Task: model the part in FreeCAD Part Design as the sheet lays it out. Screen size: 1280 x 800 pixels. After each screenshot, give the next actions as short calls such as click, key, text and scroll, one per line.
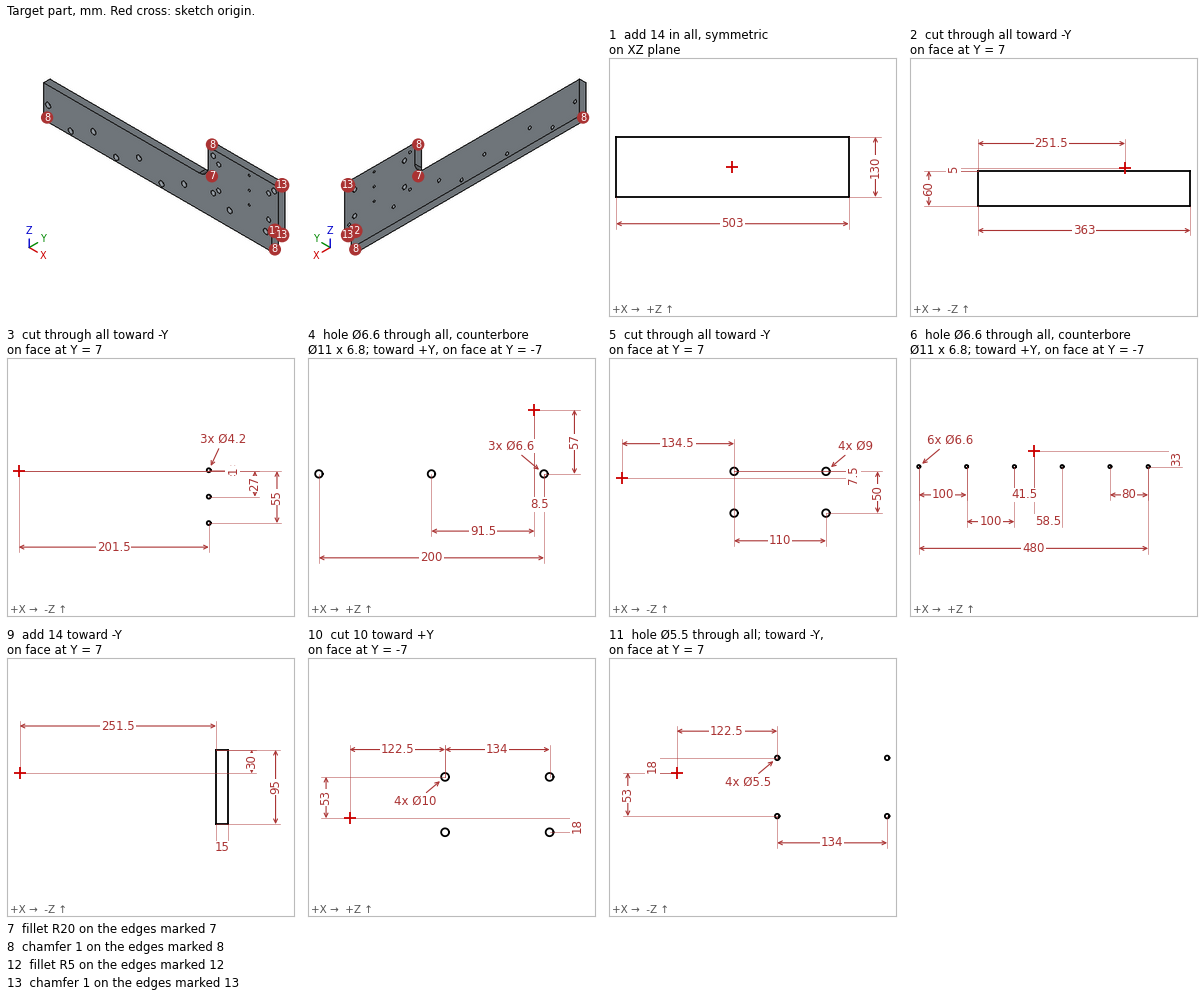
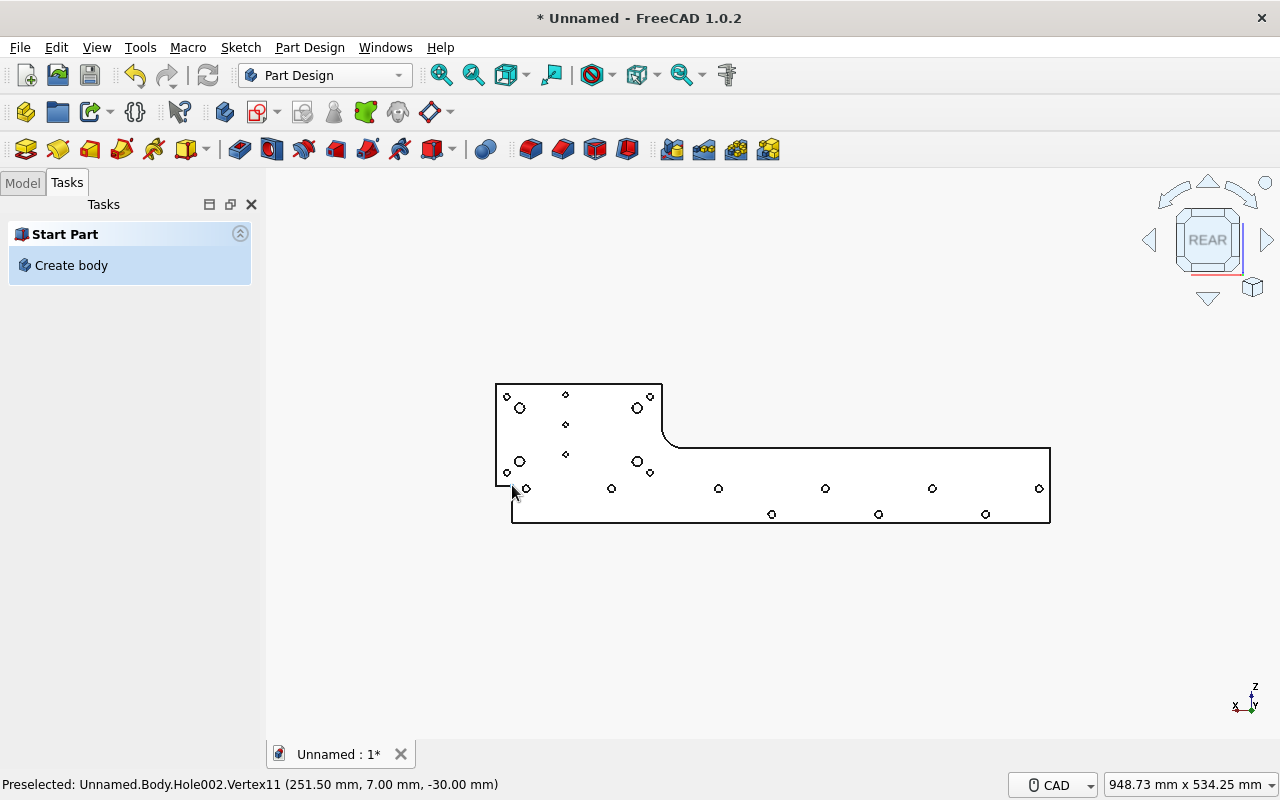
key(6)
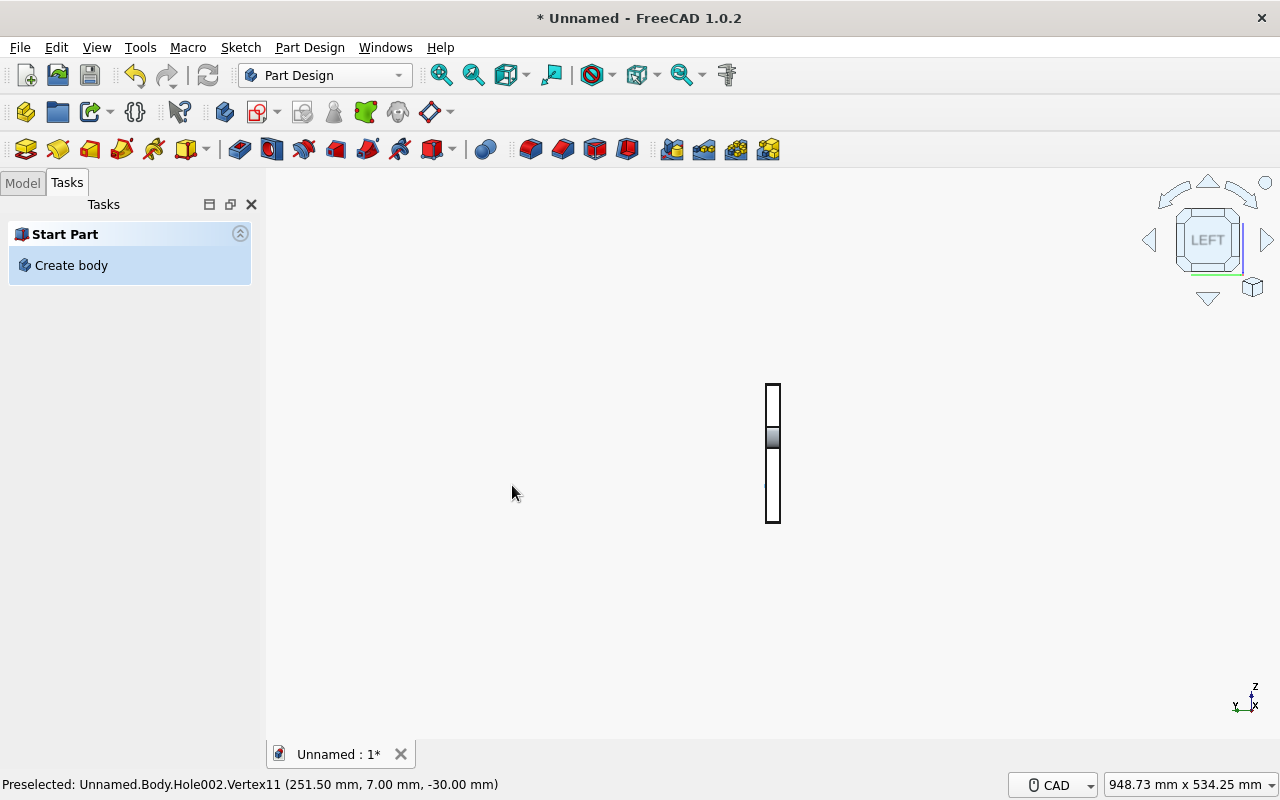
key(v)
key(f)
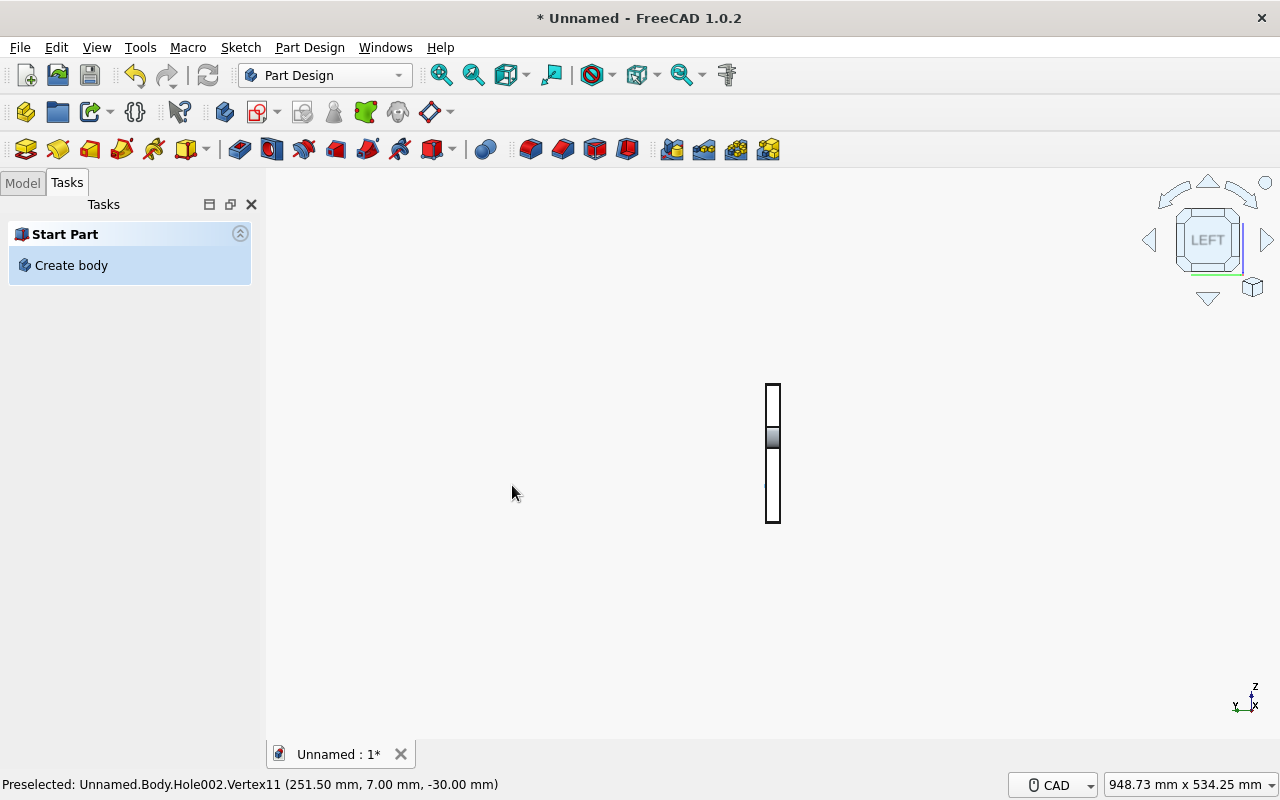
scroll(773, 485, up, 5)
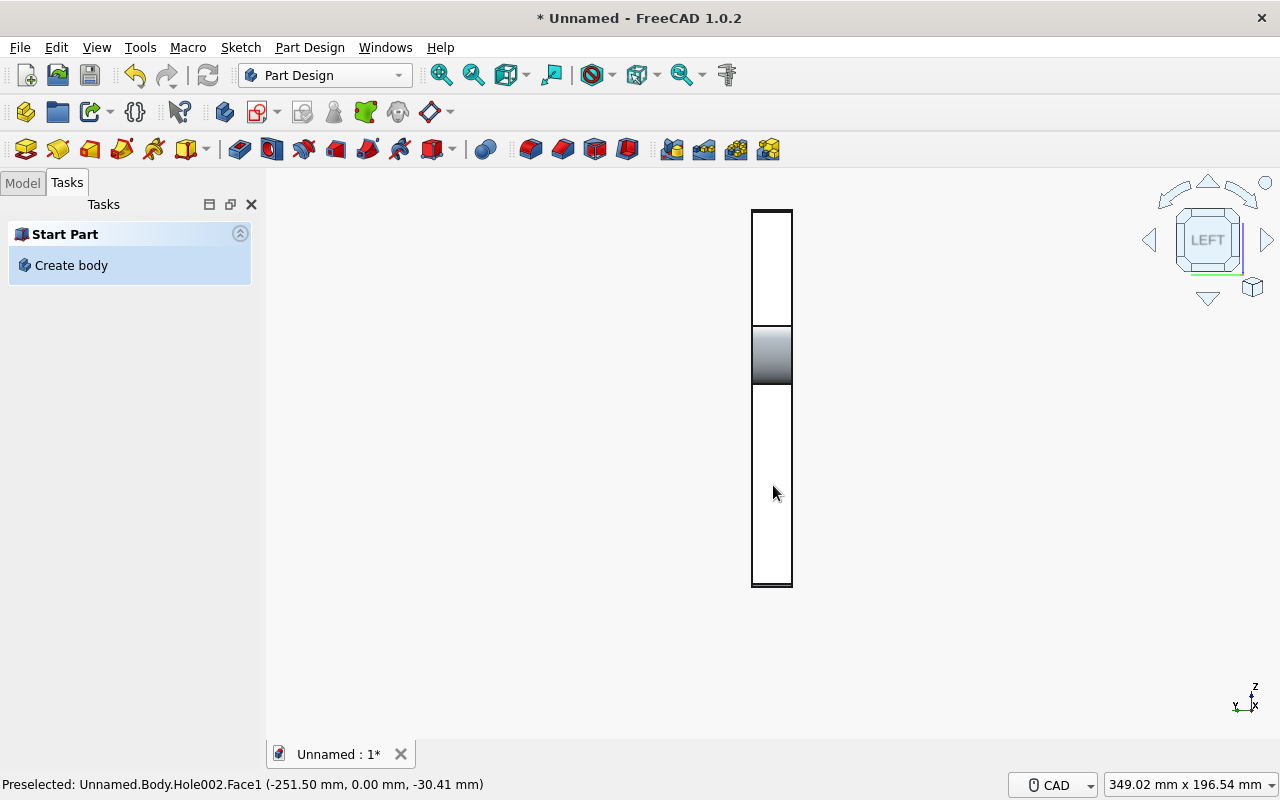
click(442, 76)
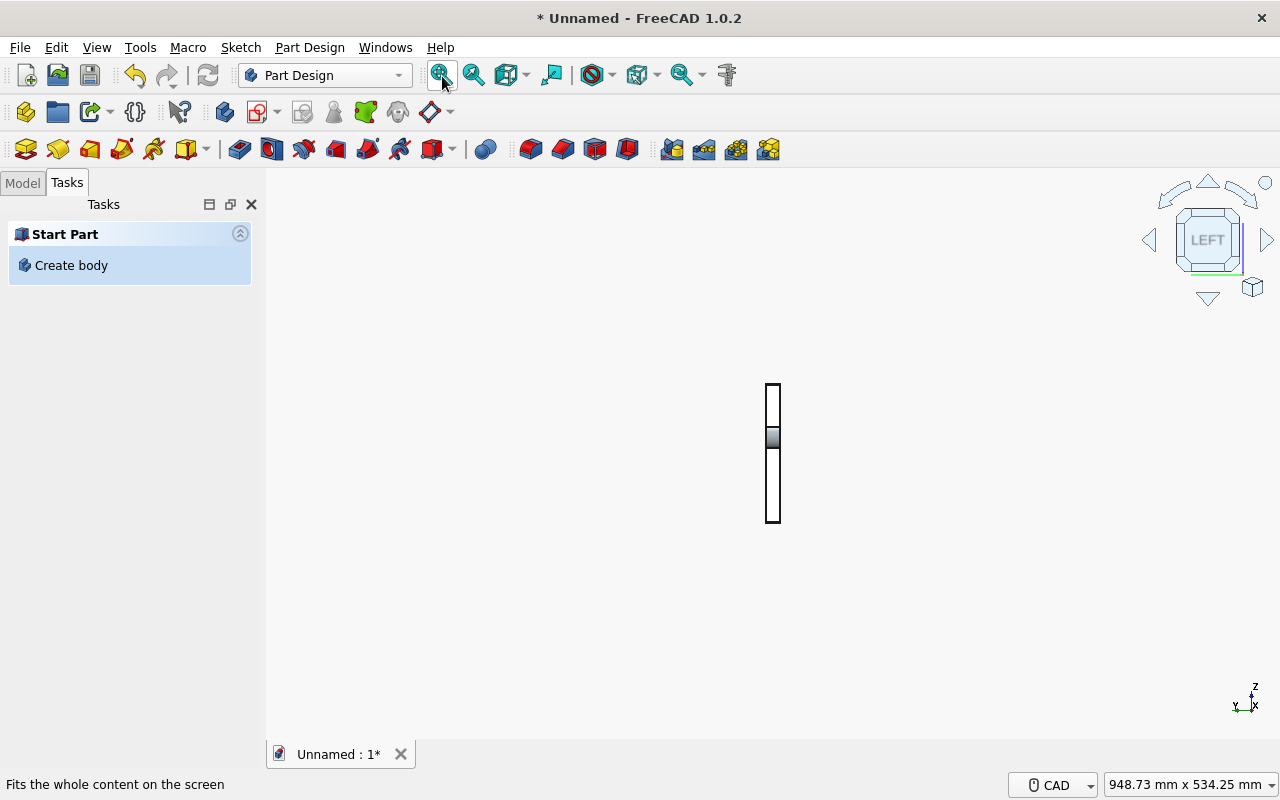
key(v)
key(3)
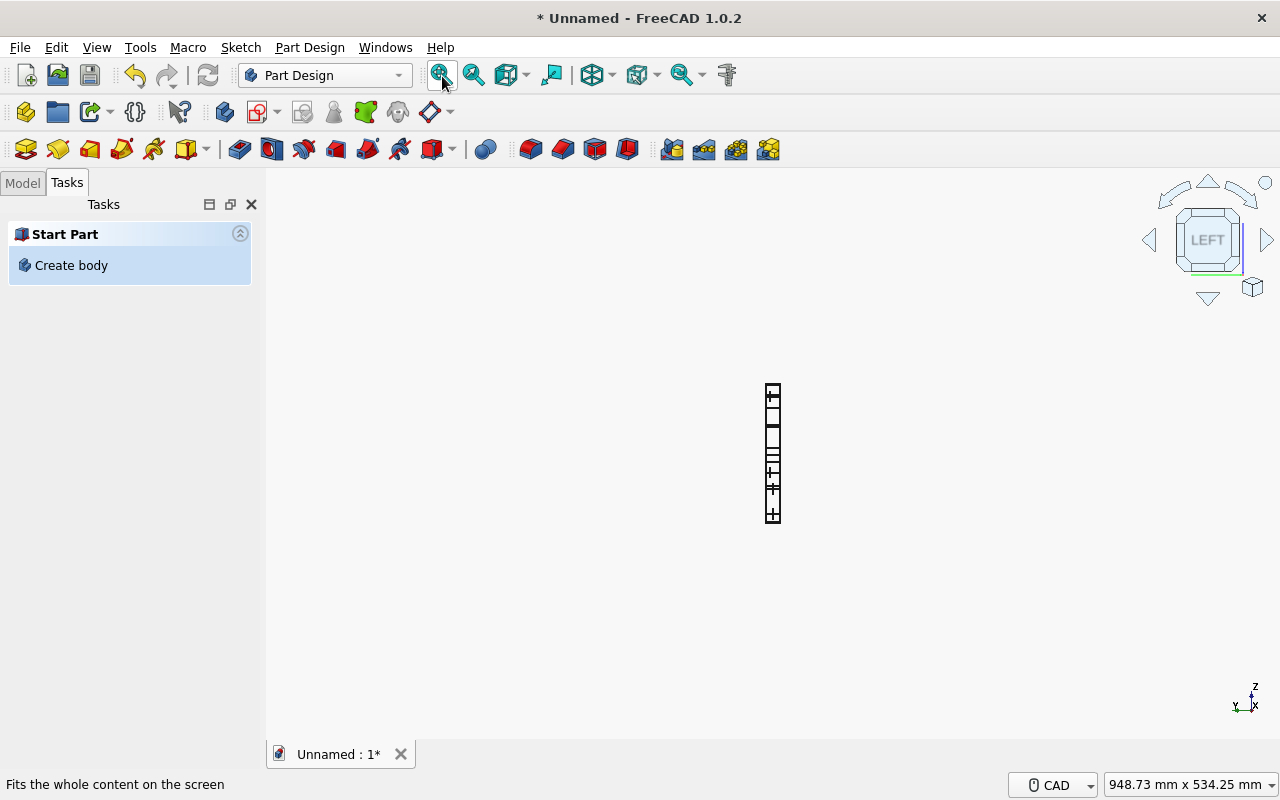
key(0)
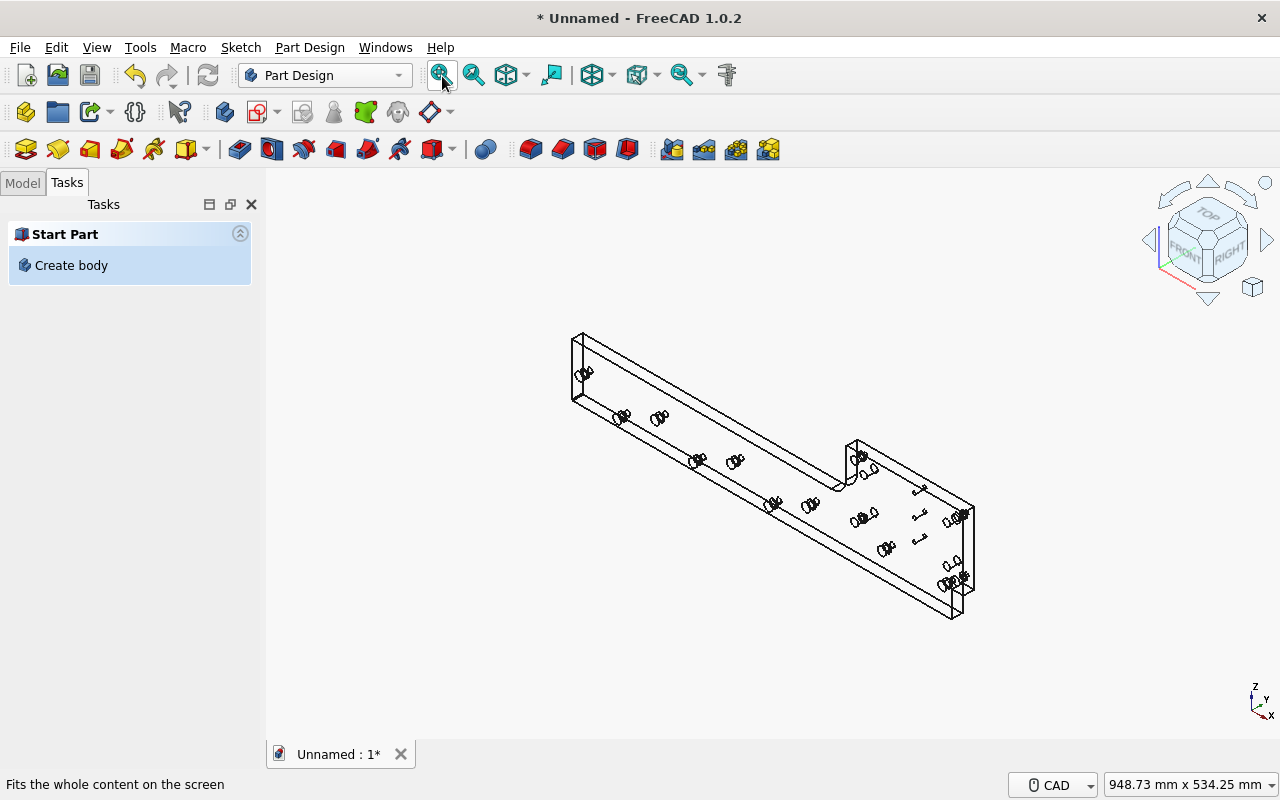
scroll(957, 585, up, 6)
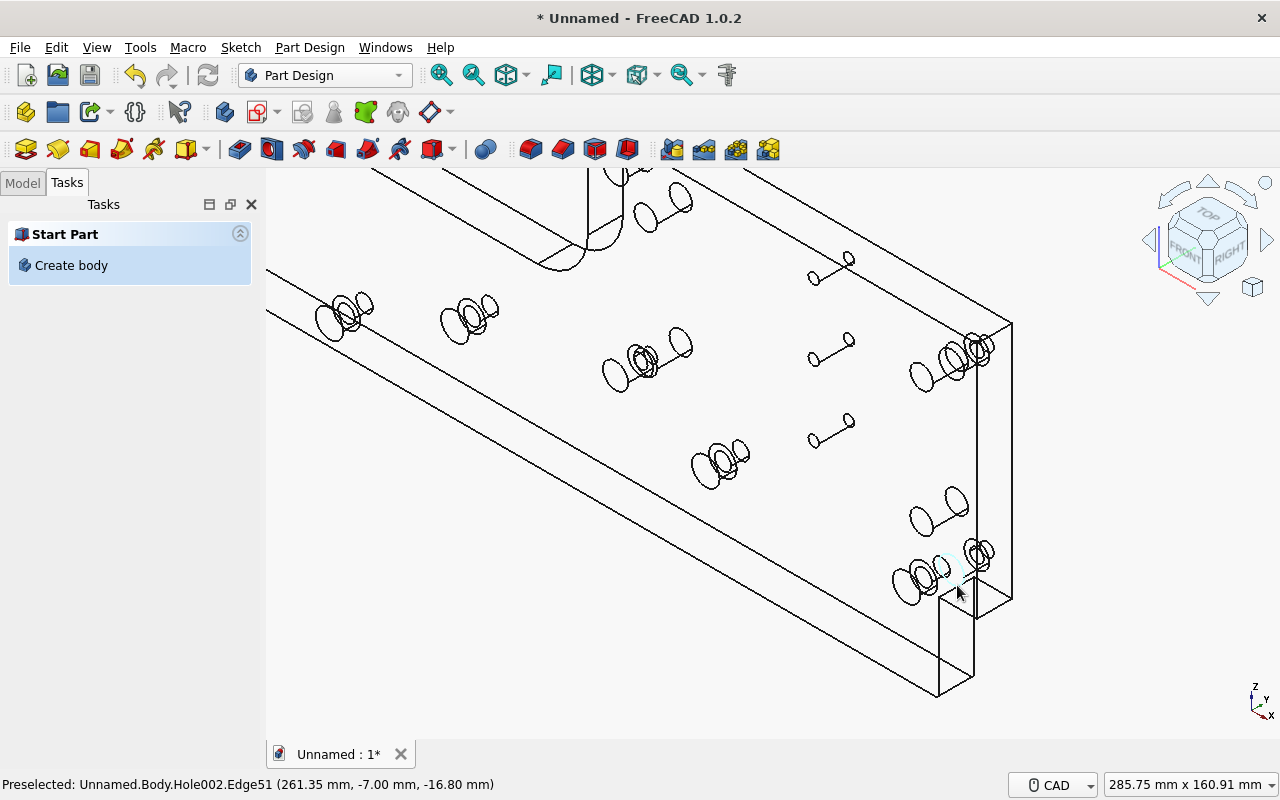
click(950, 590)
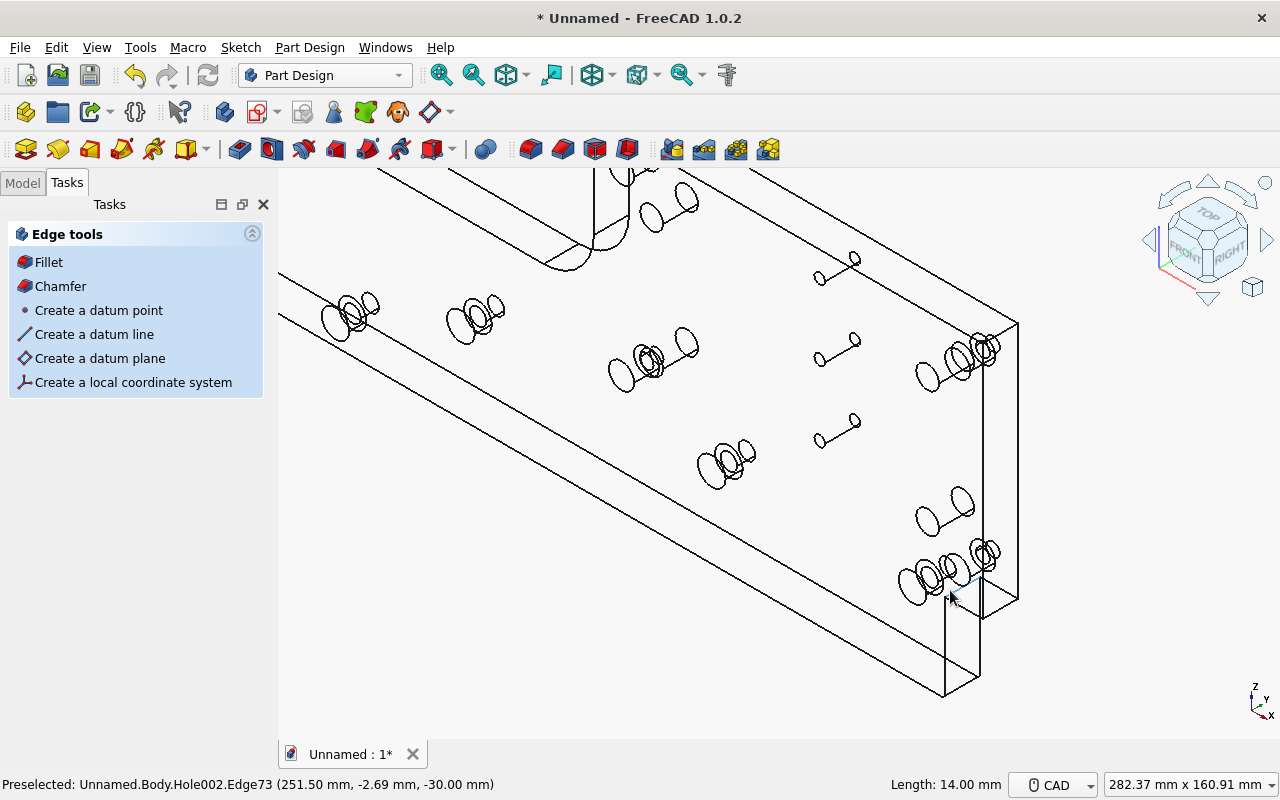
key(v)
key(1)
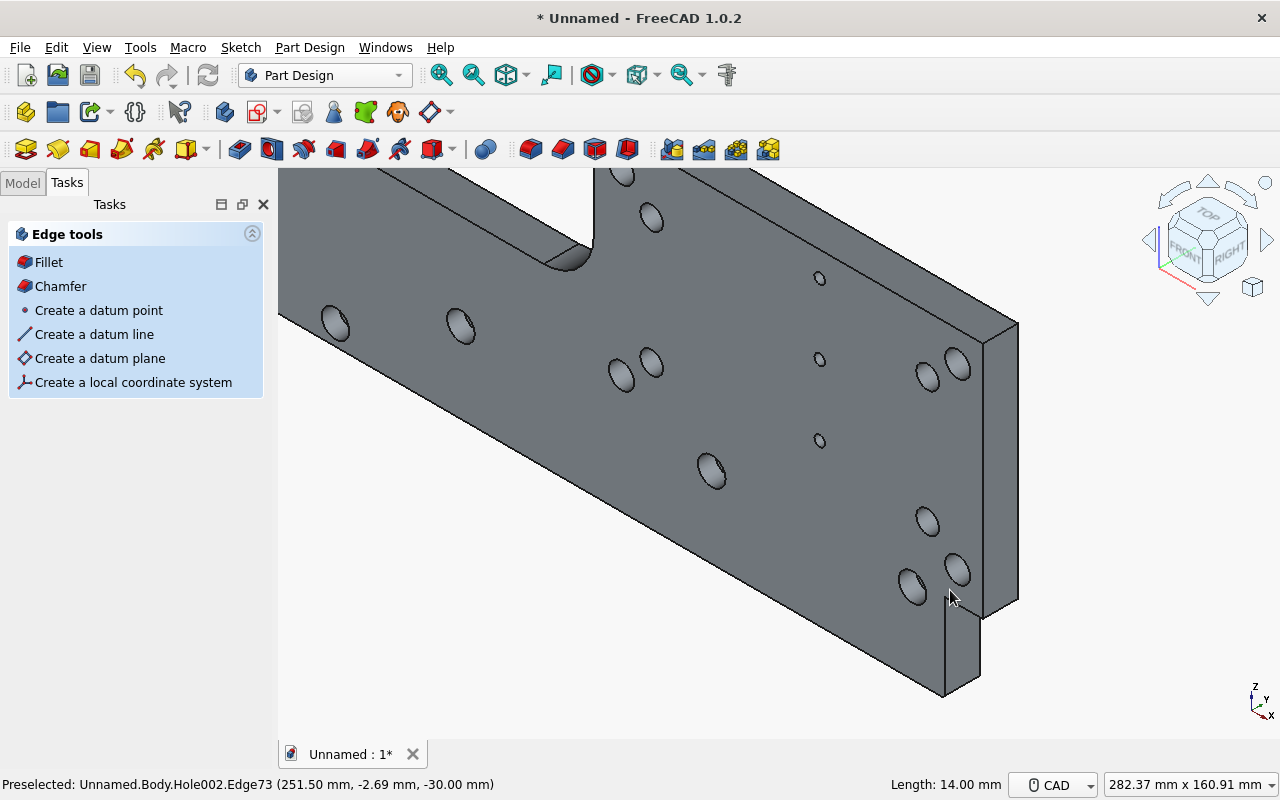
click(532, 150)